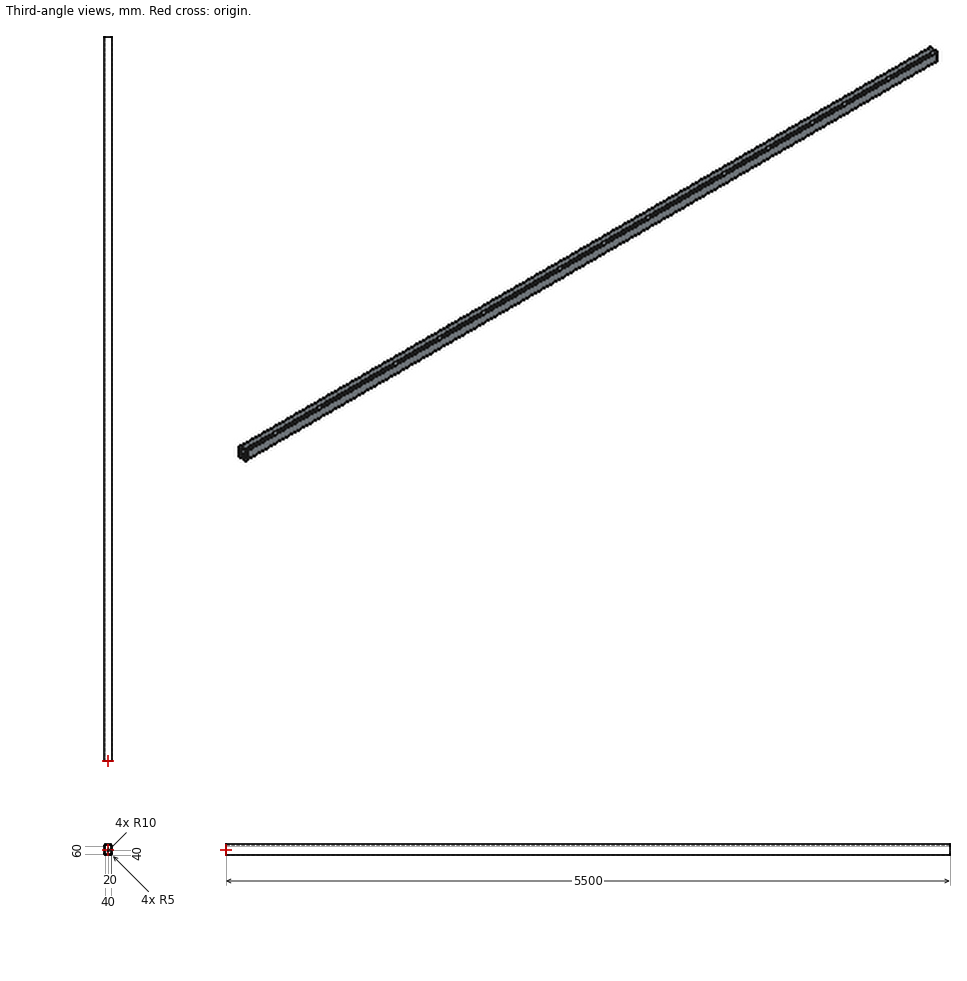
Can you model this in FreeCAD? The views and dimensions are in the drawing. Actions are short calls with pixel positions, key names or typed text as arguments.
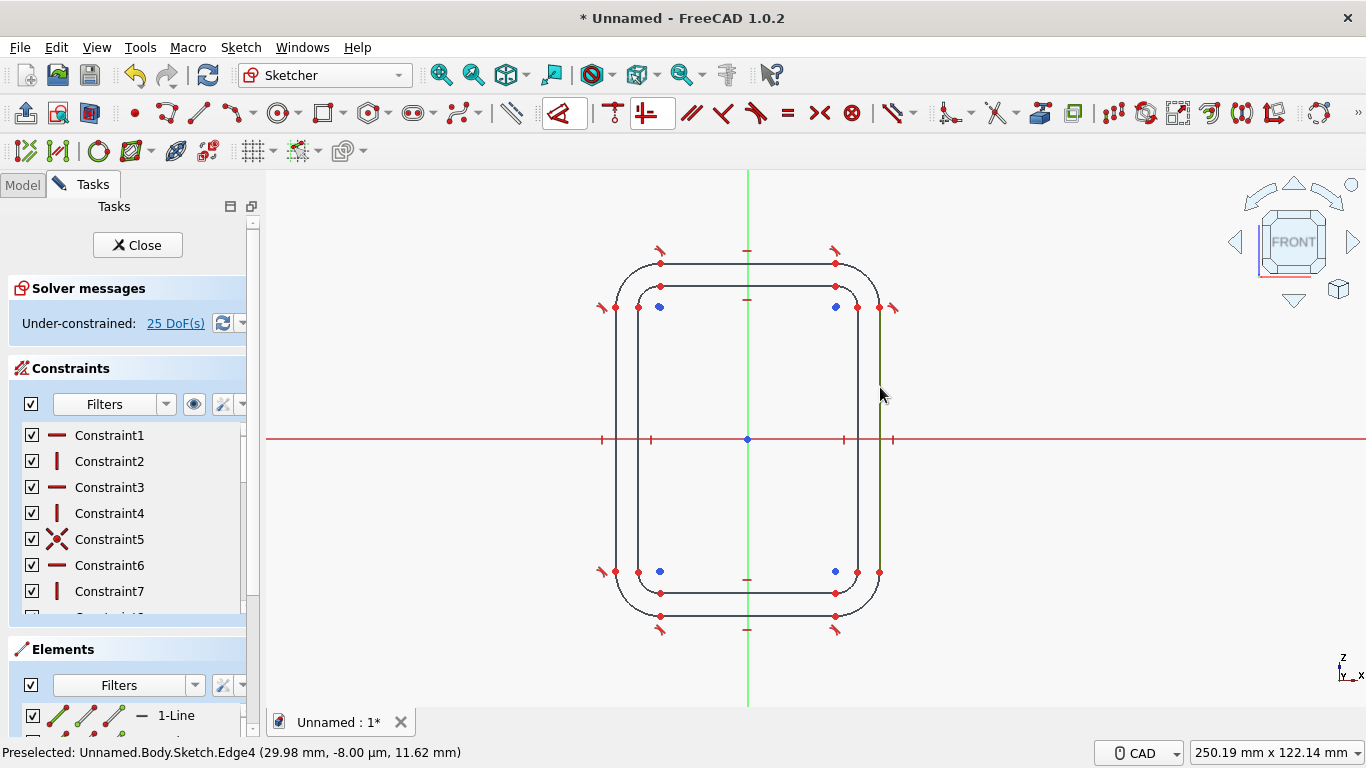
click(855, 611)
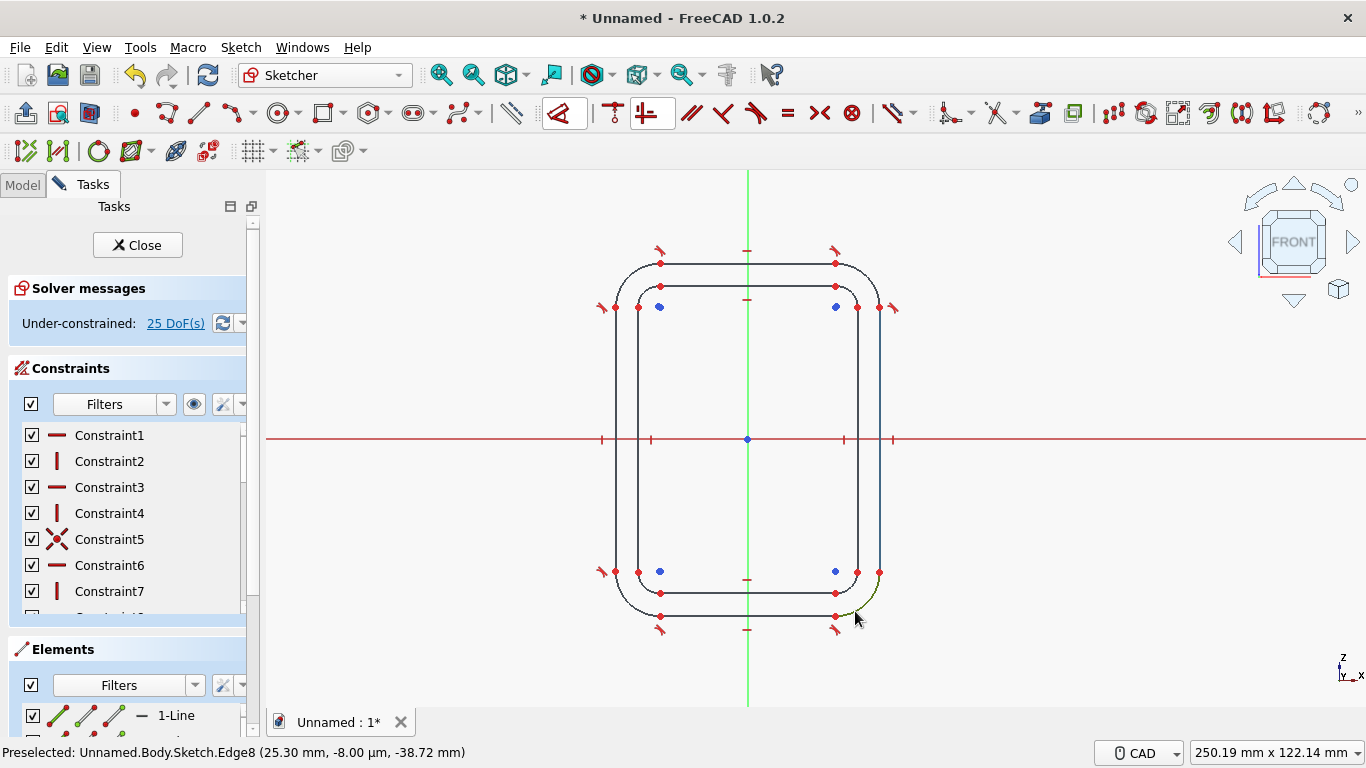
click(756, 114)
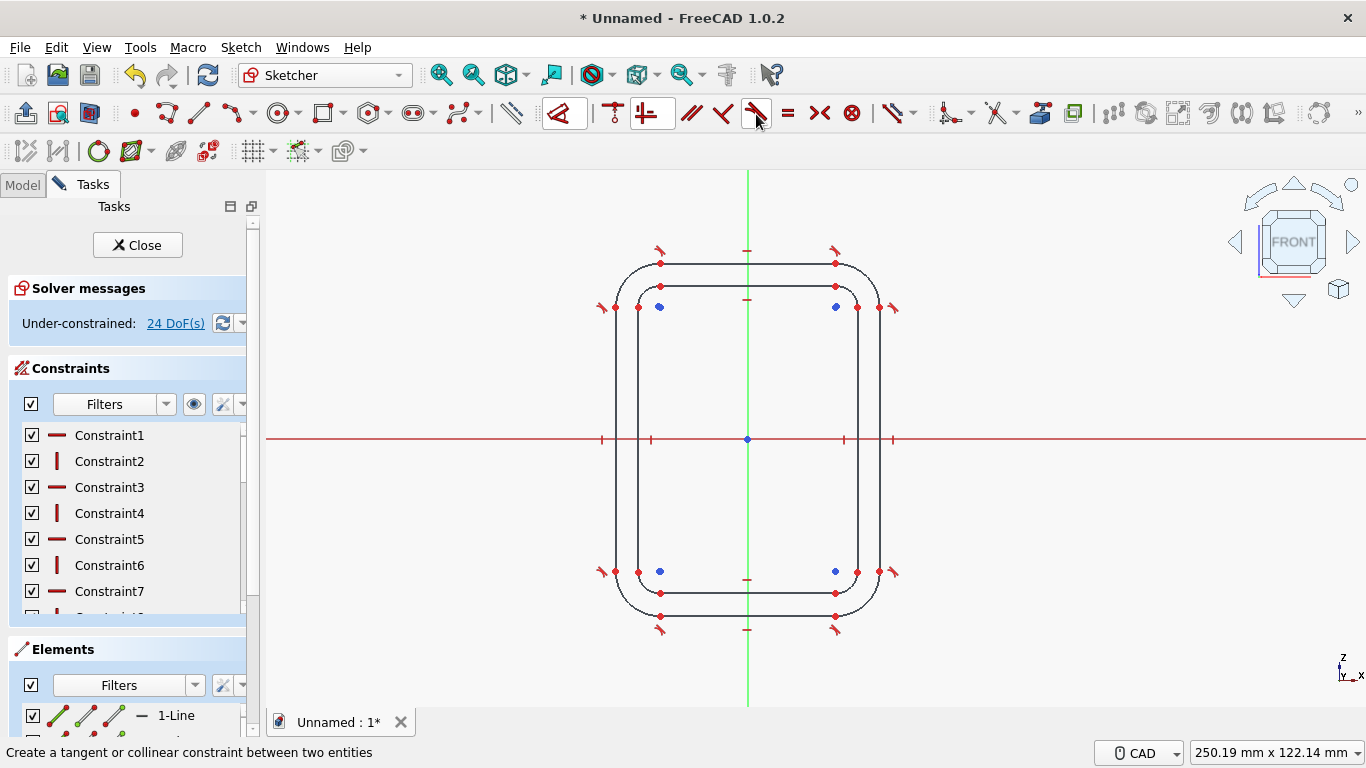
click(713, 593)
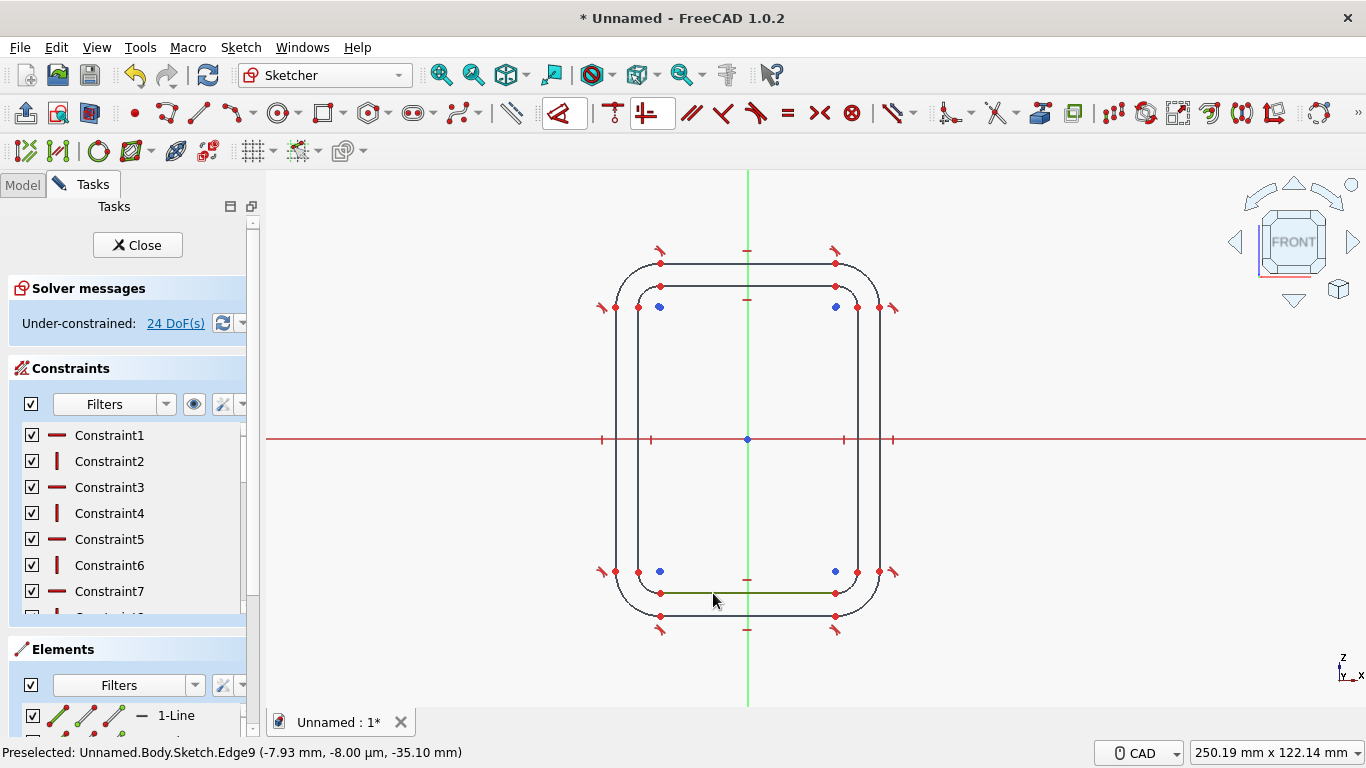
scroll(845, 591, up, 2)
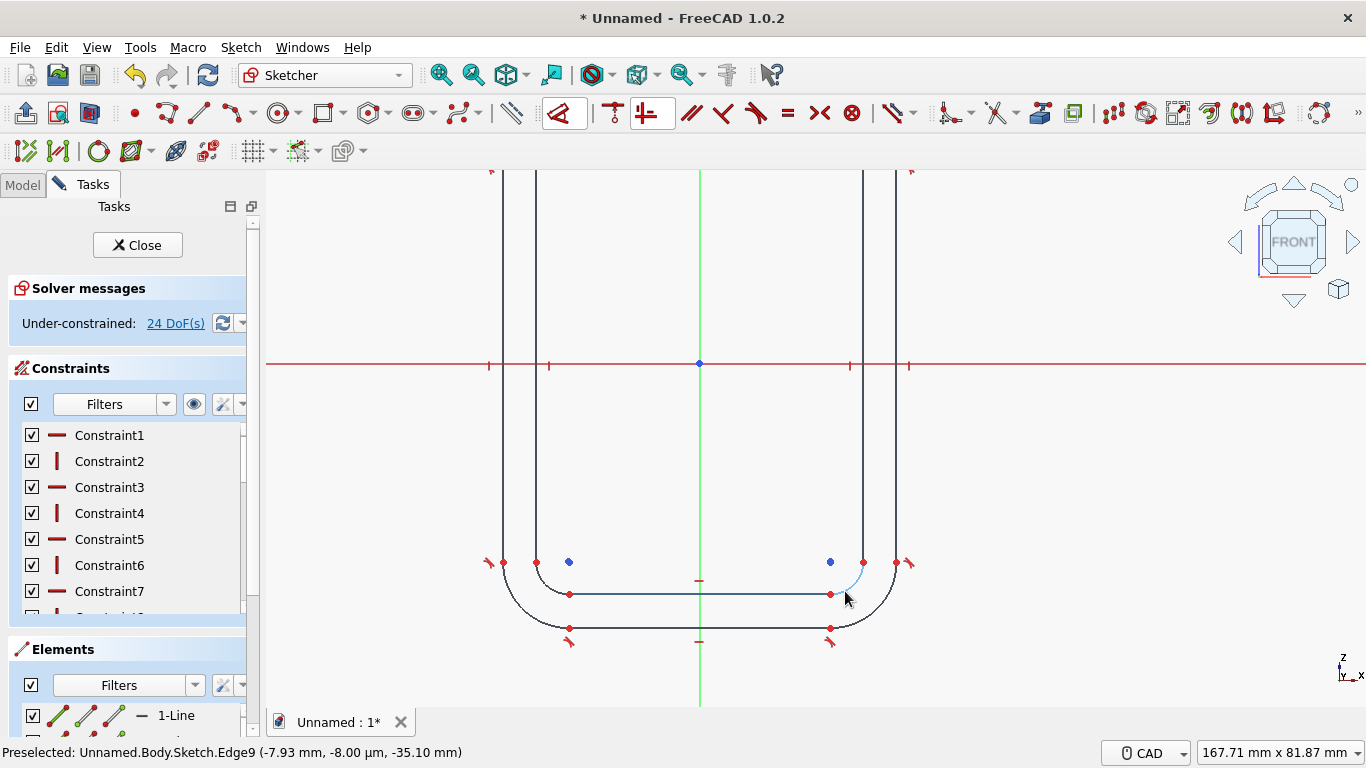
click(845, 591)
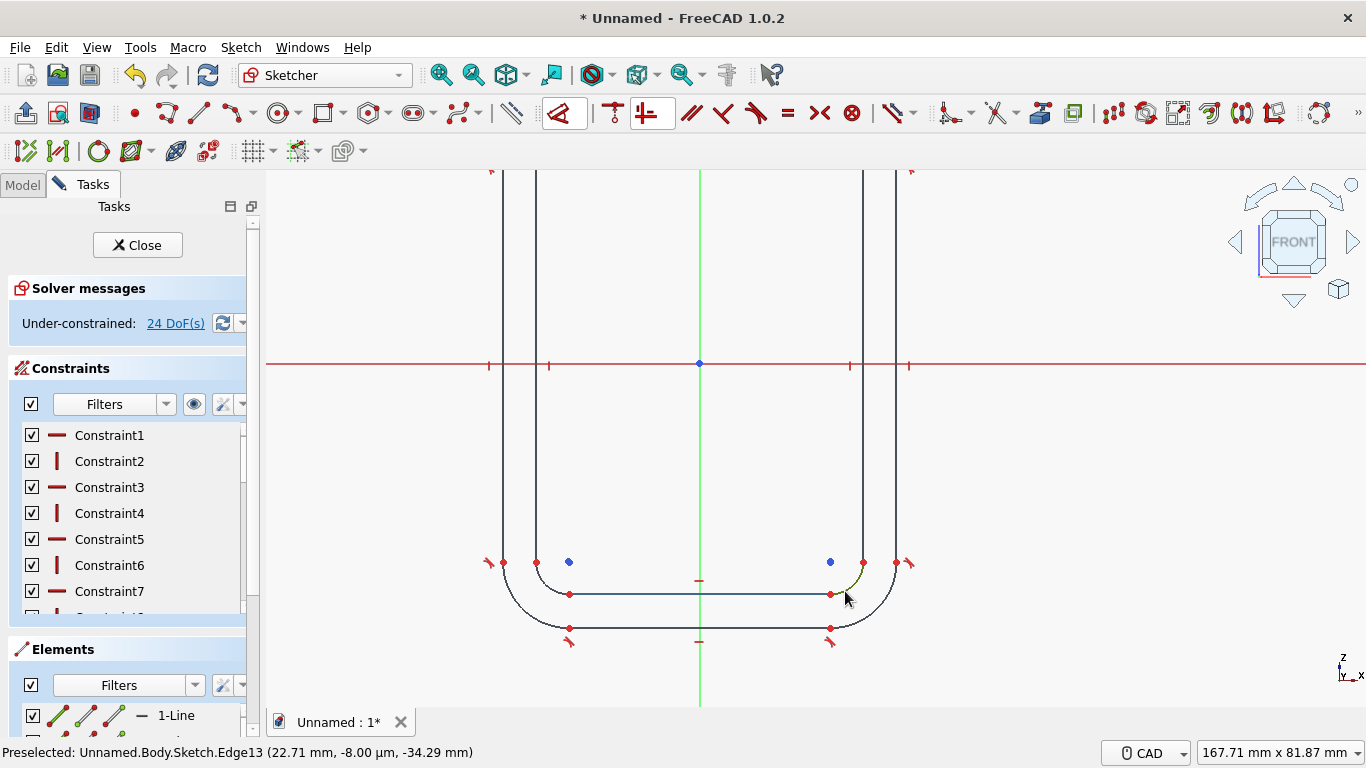
click(756, 114)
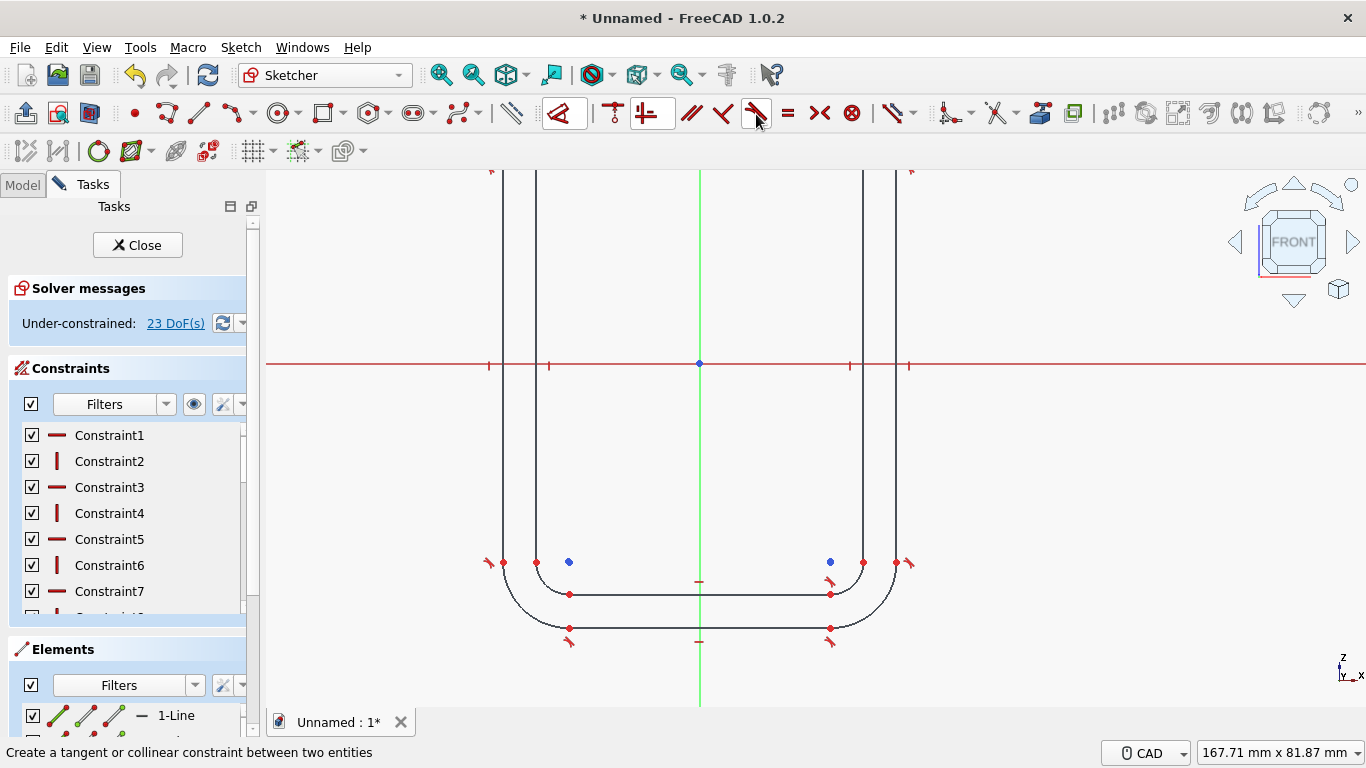
click(648, 595)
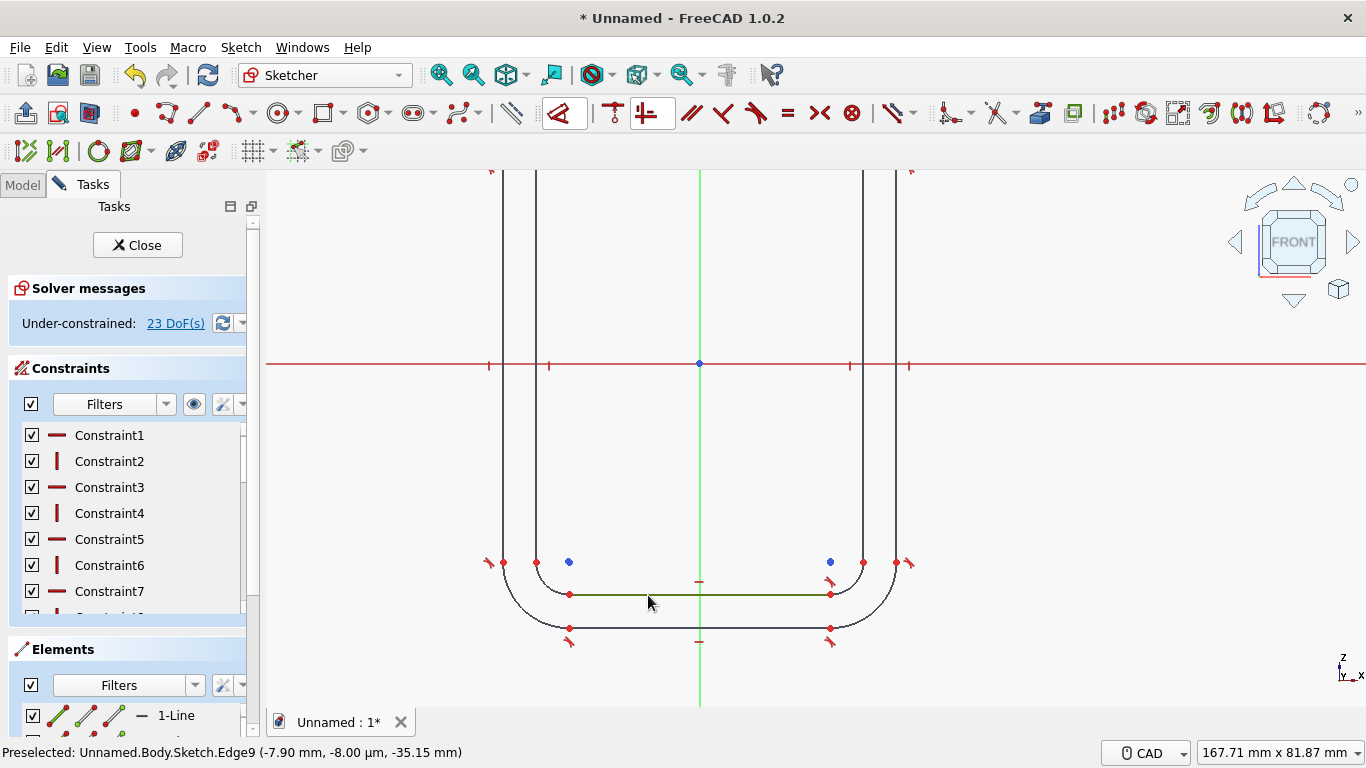
click(540, 577)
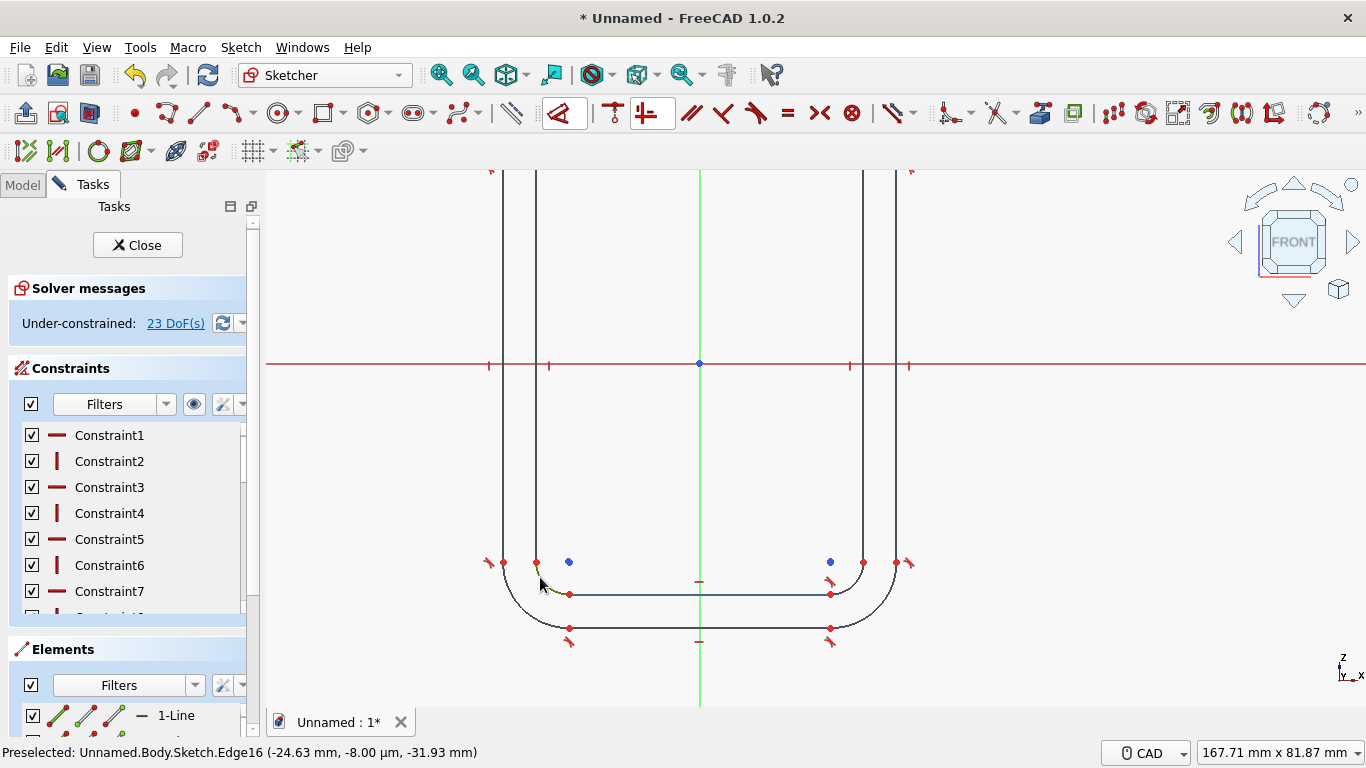
click(756, 114)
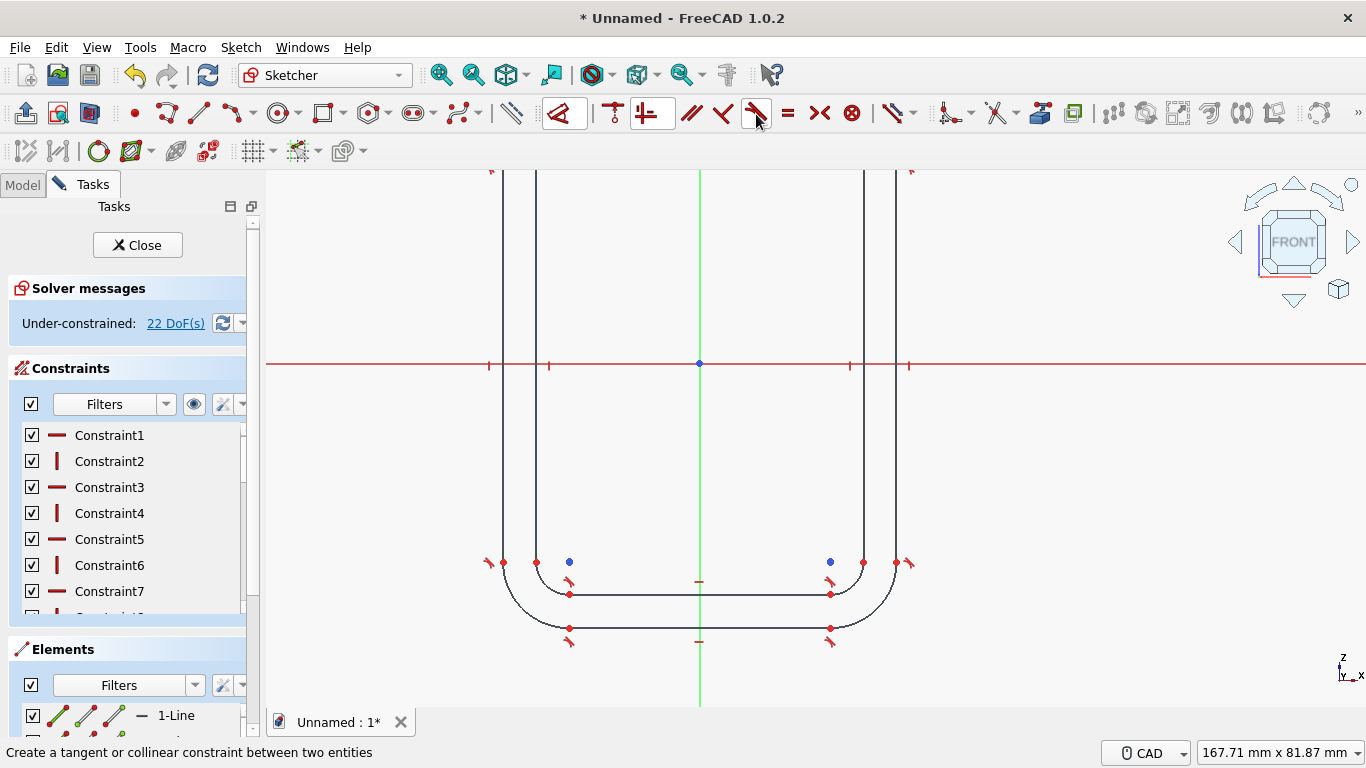
click(864, 444)